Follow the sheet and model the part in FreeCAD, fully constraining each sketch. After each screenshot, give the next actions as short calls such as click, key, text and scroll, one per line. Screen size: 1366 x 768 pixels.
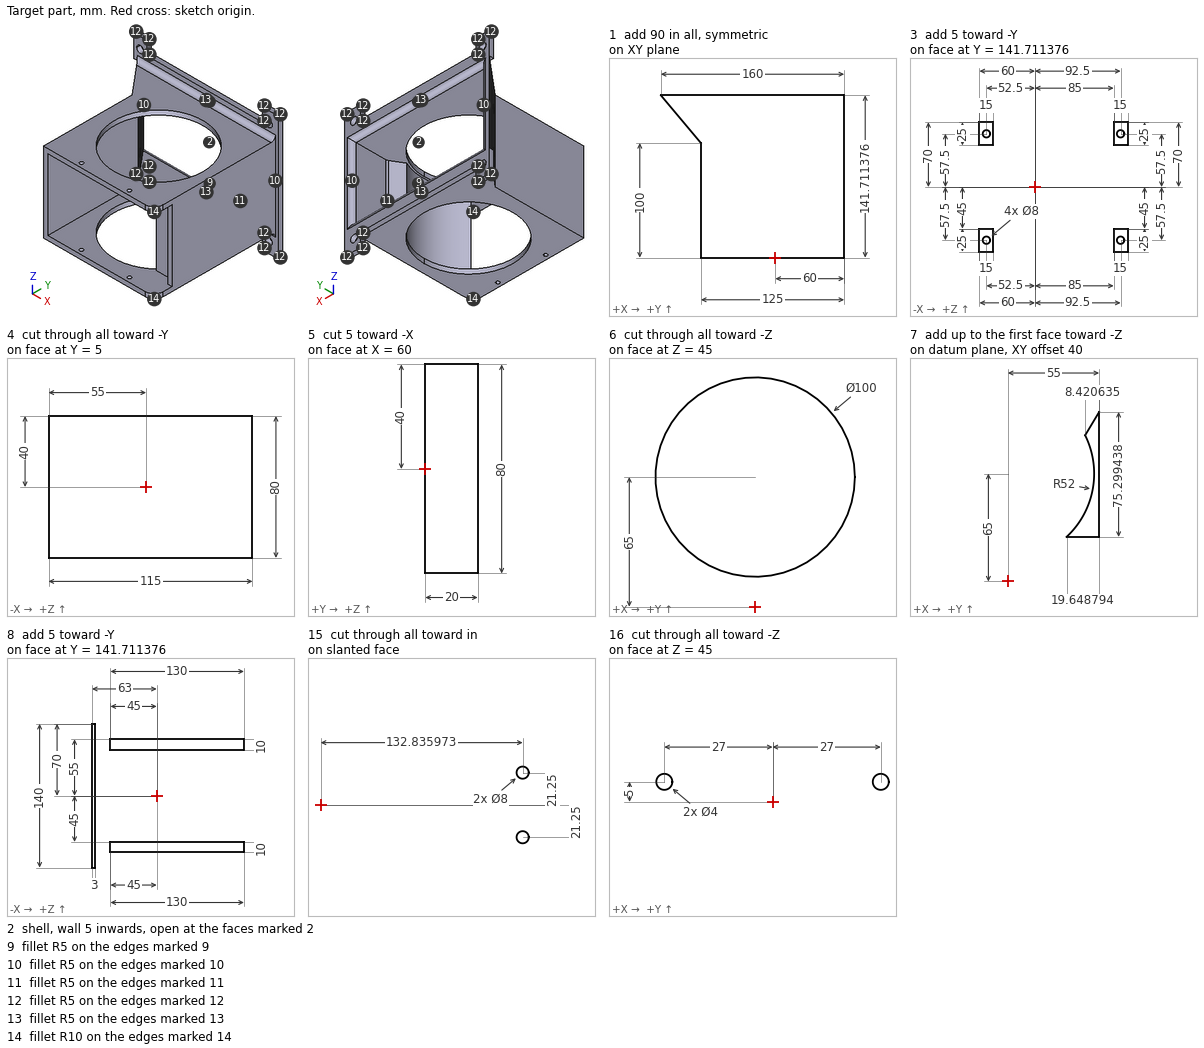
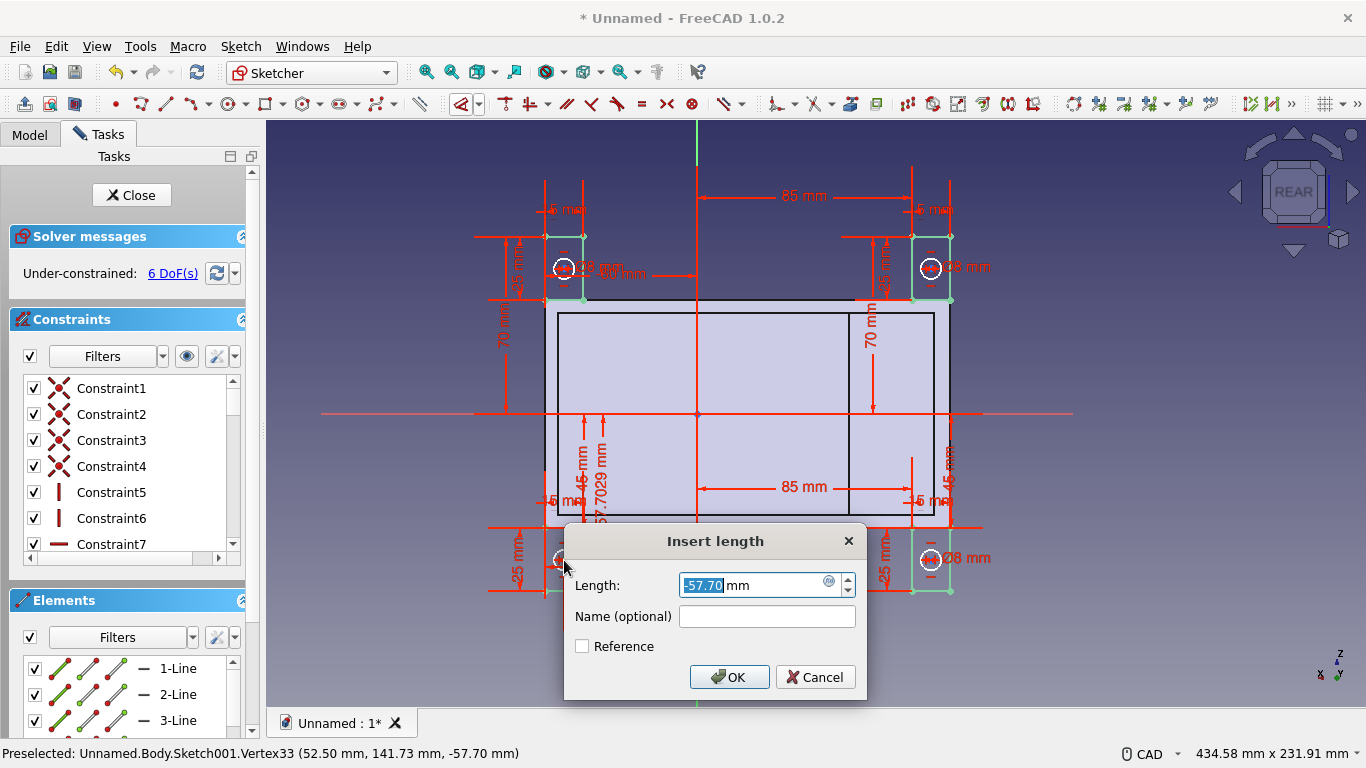
text(-57.5)
key(Return)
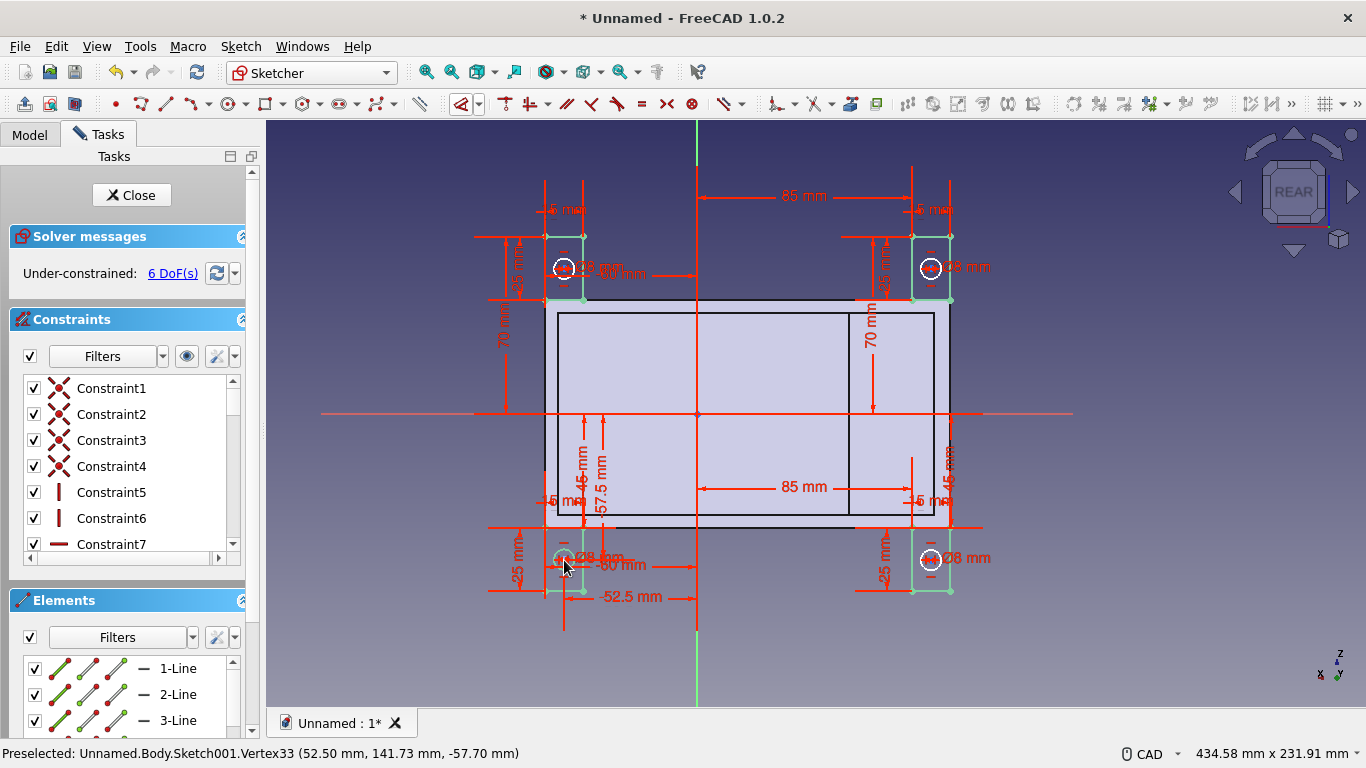
click(931, 269)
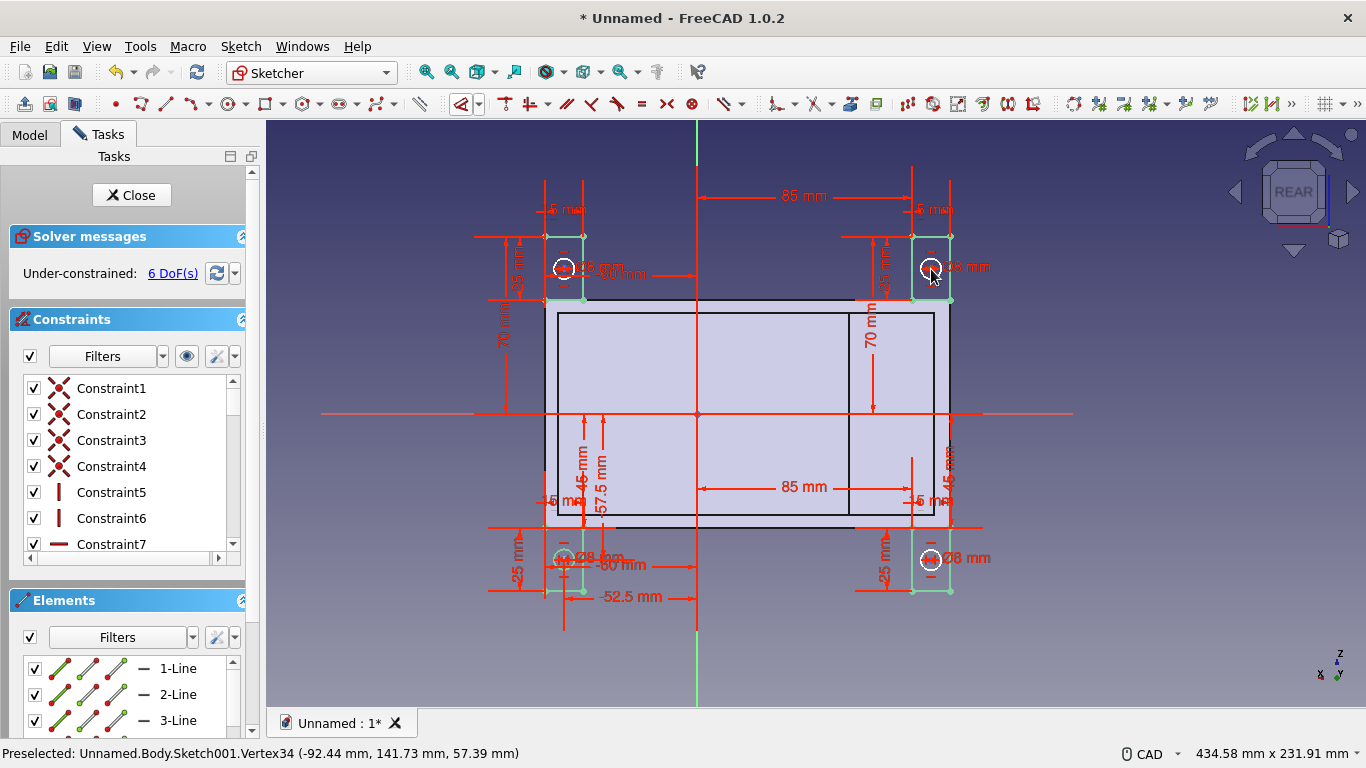
key(l)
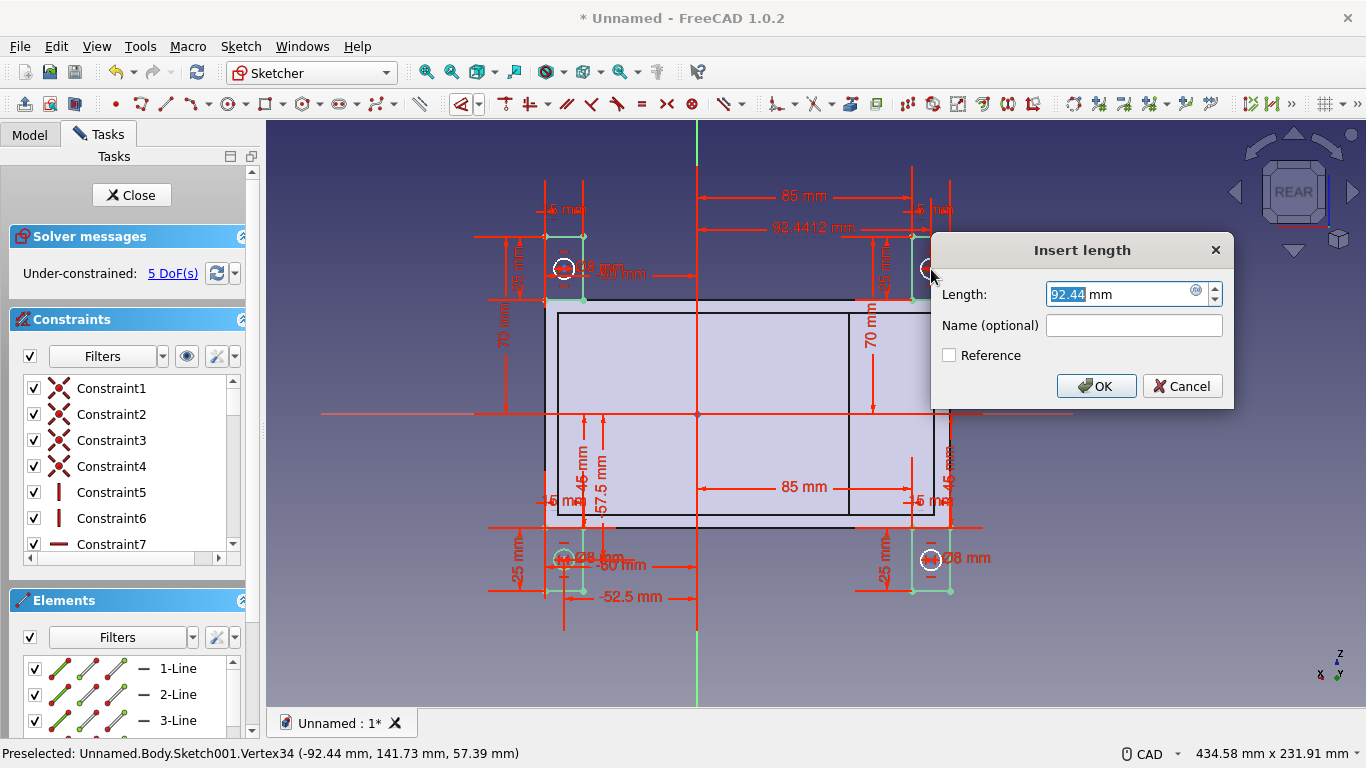
text(92.5)
key(Return)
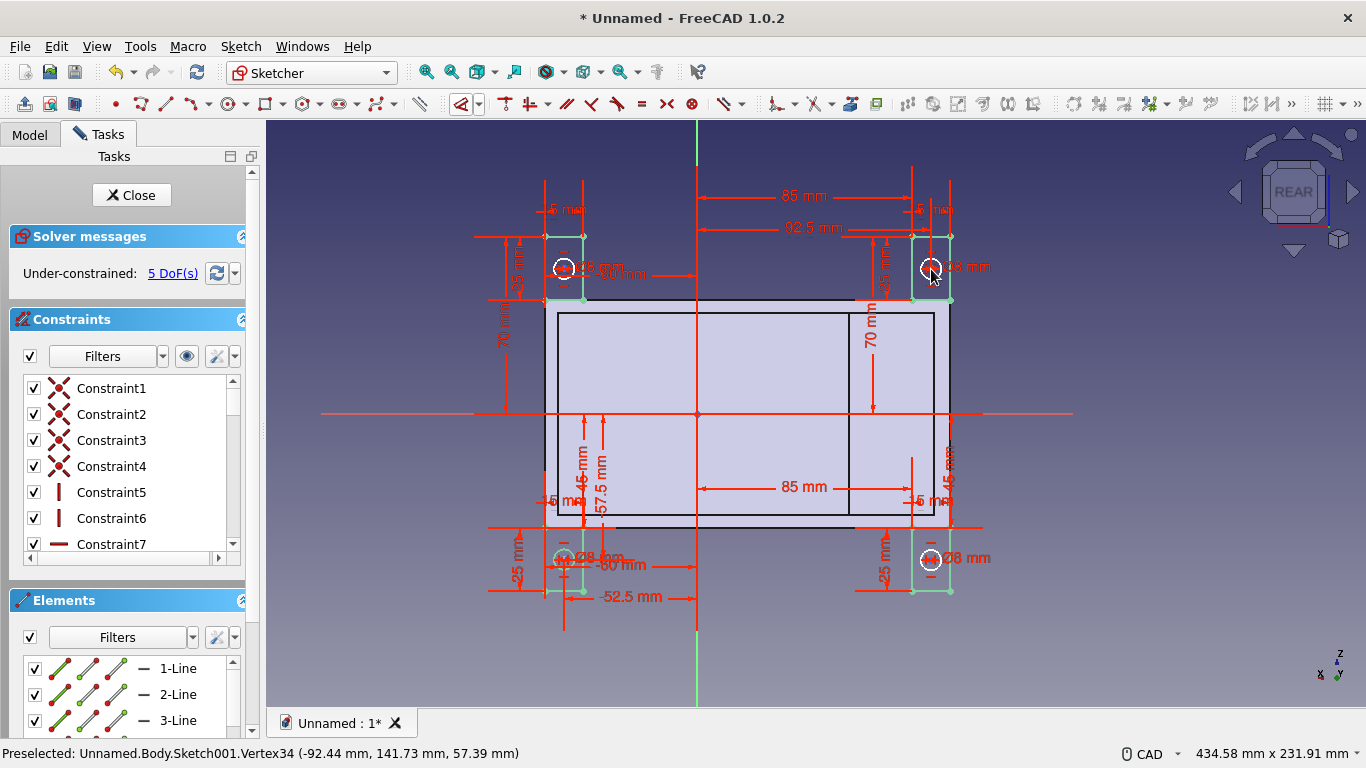
click(931, 269)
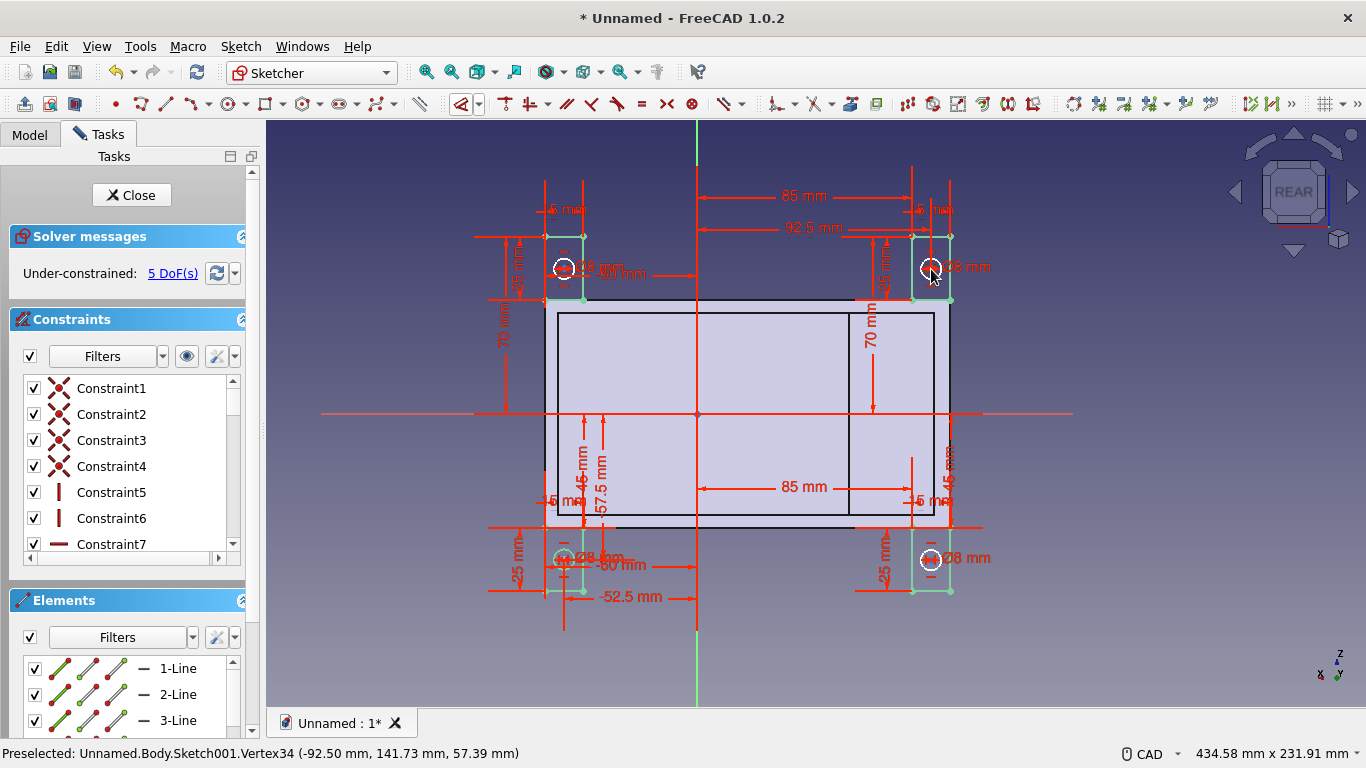
key(i)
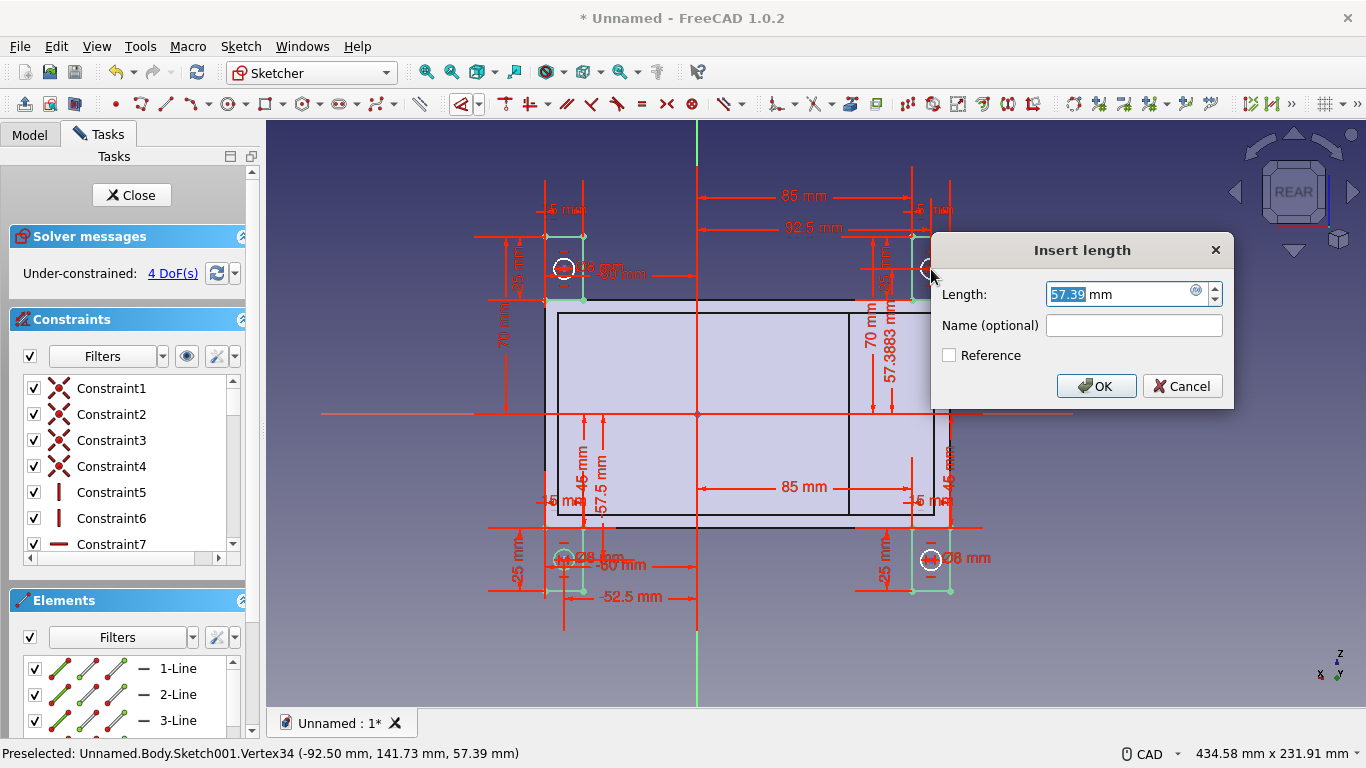
text(57.5)
key(Return)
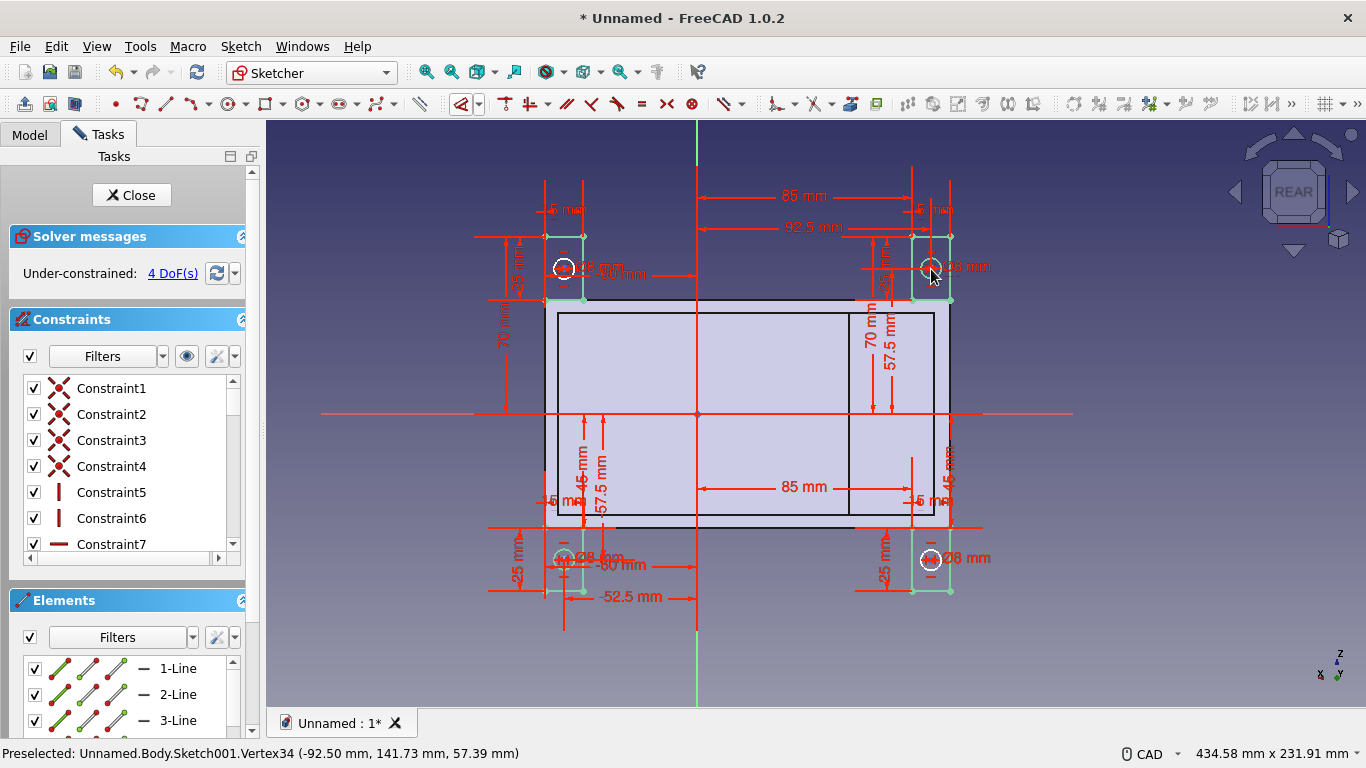
click(564, 269)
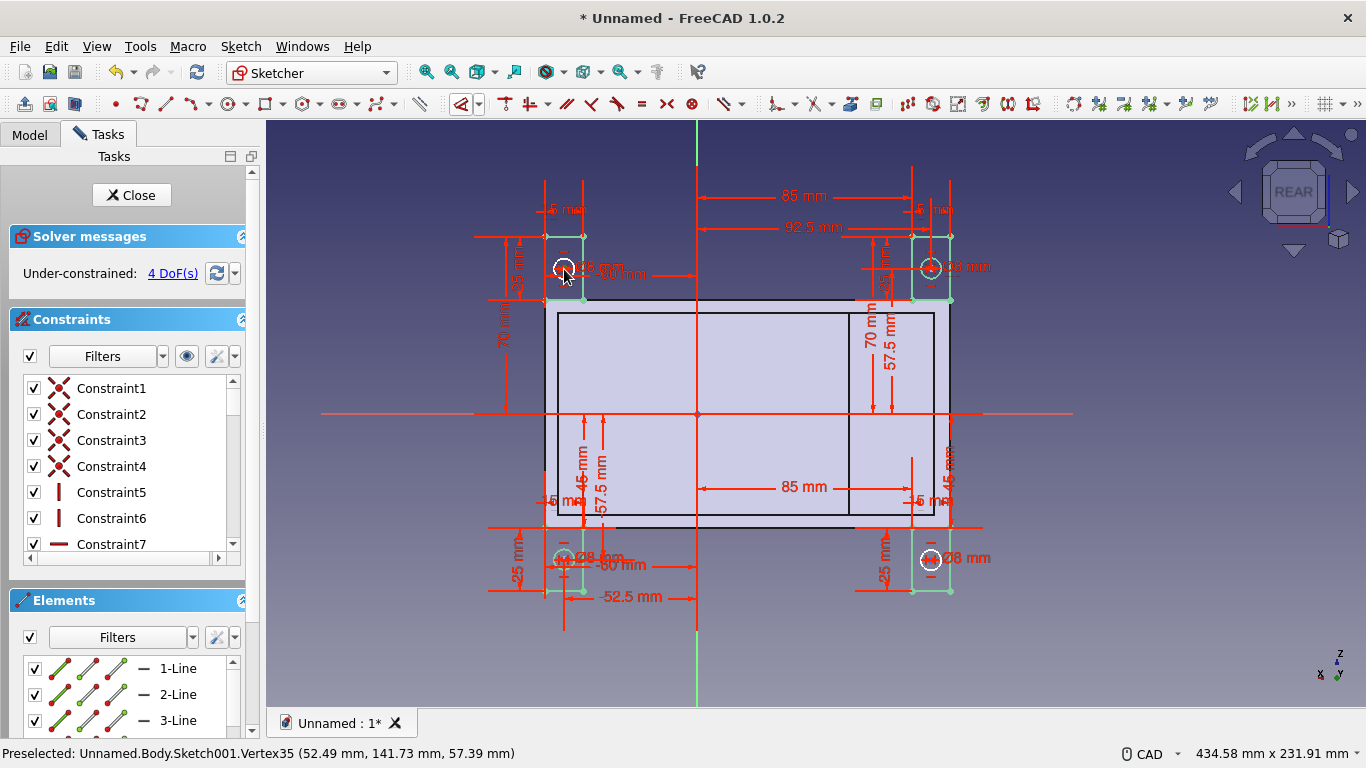
click(478, 104)